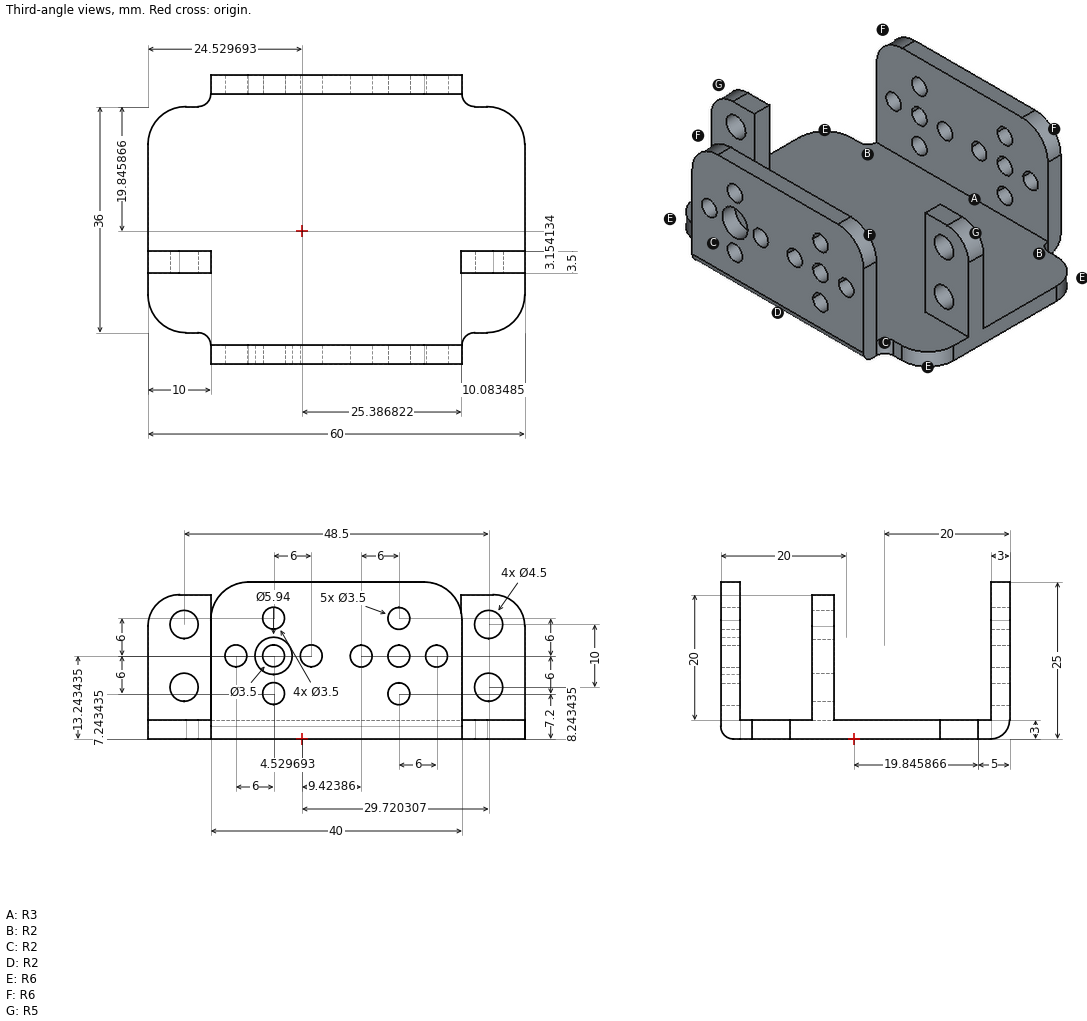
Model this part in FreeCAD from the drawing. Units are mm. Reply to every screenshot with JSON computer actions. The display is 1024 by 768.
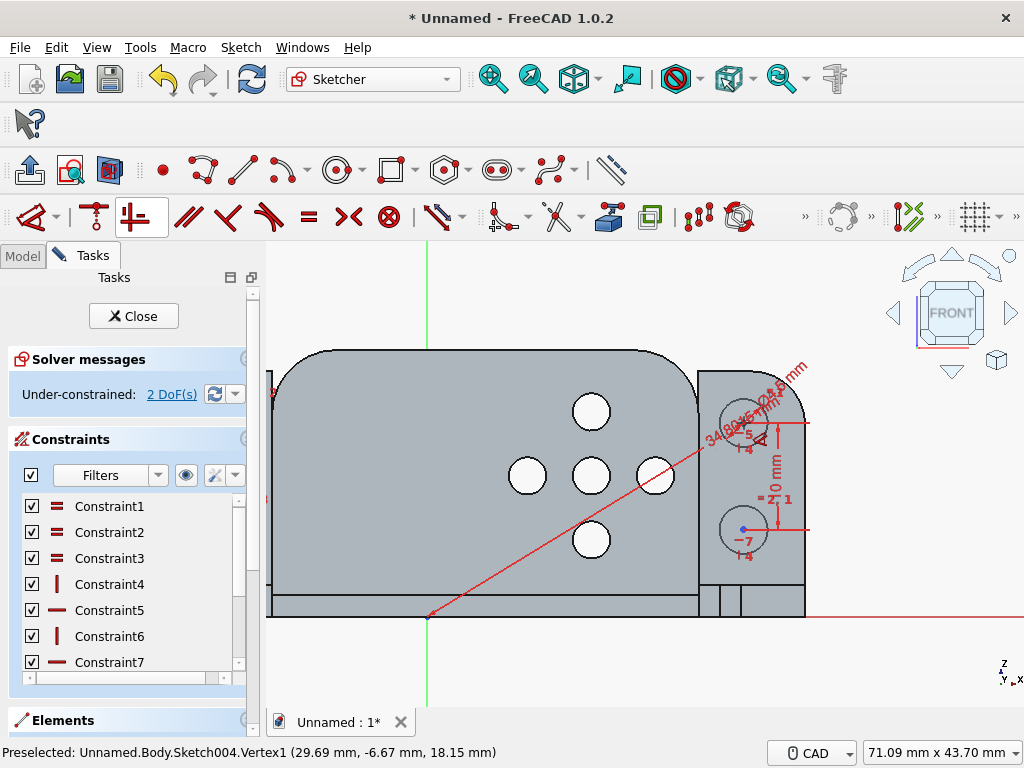
{"action": "scroll", "coordinate": [762, 406], "scroll_direction": "down", "scroll_amount": 2}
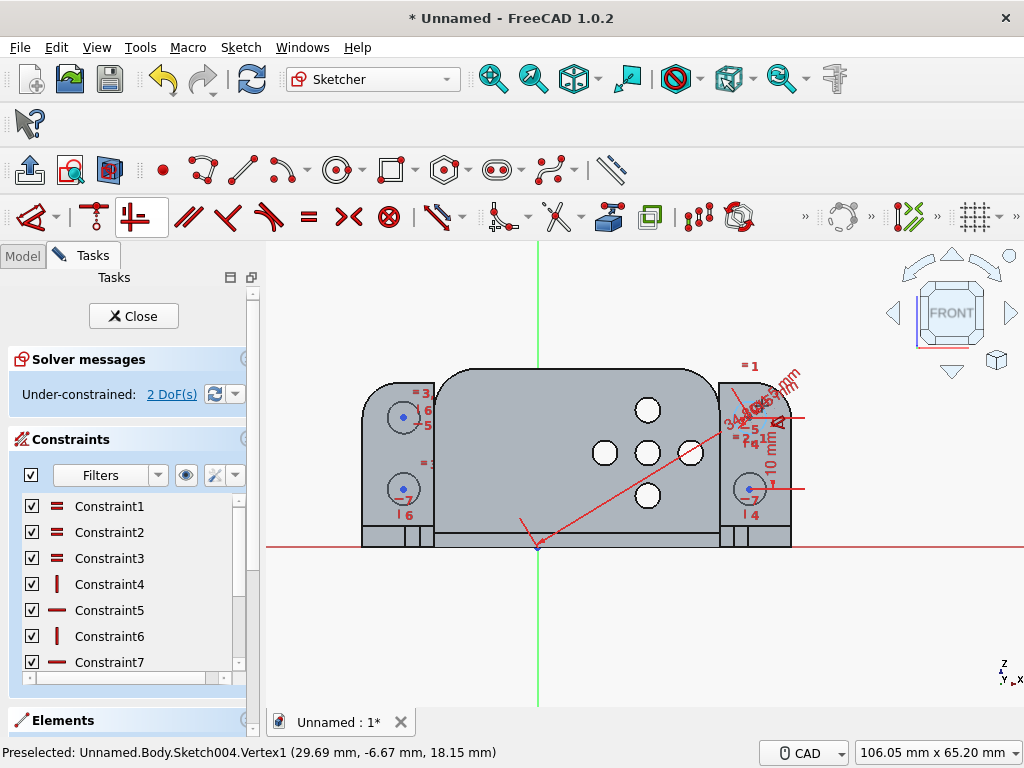
{"action": "left_click", "coordinate": [404, 418]}
{"action": "left_click", "coordinate": [577, 384]}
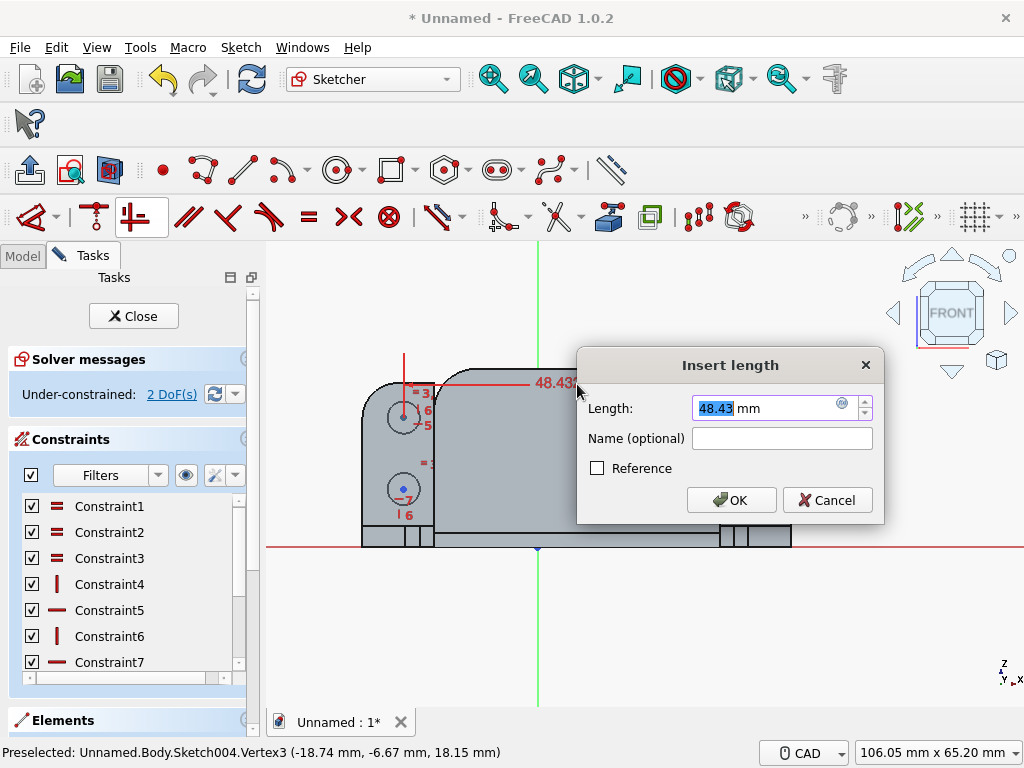
{"action": "type", "text": "48.5"}
{"action": "key", "text": "Return"}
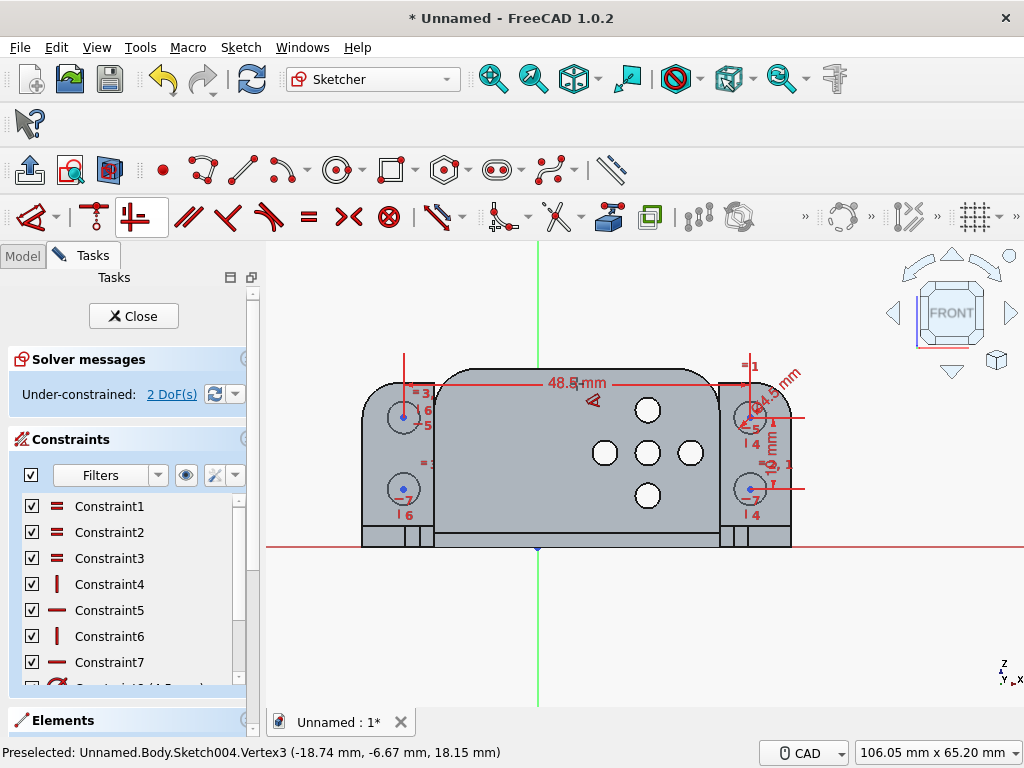
{"action": "left_click", "coordinate": [750, 489]}
{"action": "left_click", "coordinate": [784, 518]}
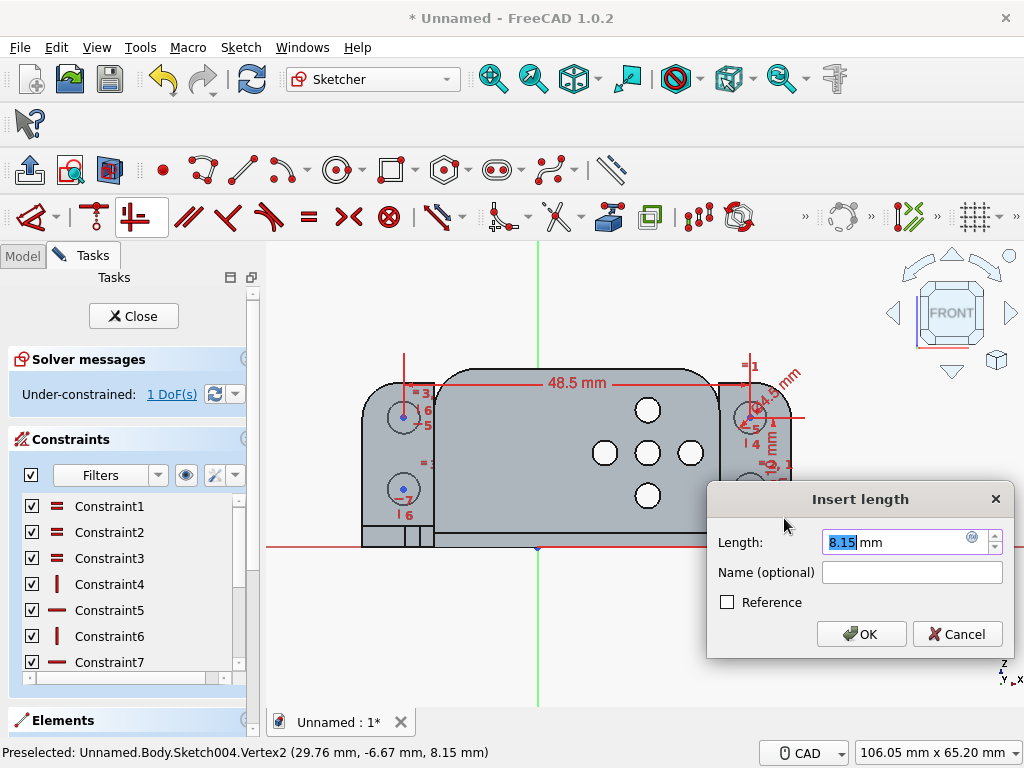
{"action": "type", "text": "8.243435"}
{"action": "key", "text": "Return"}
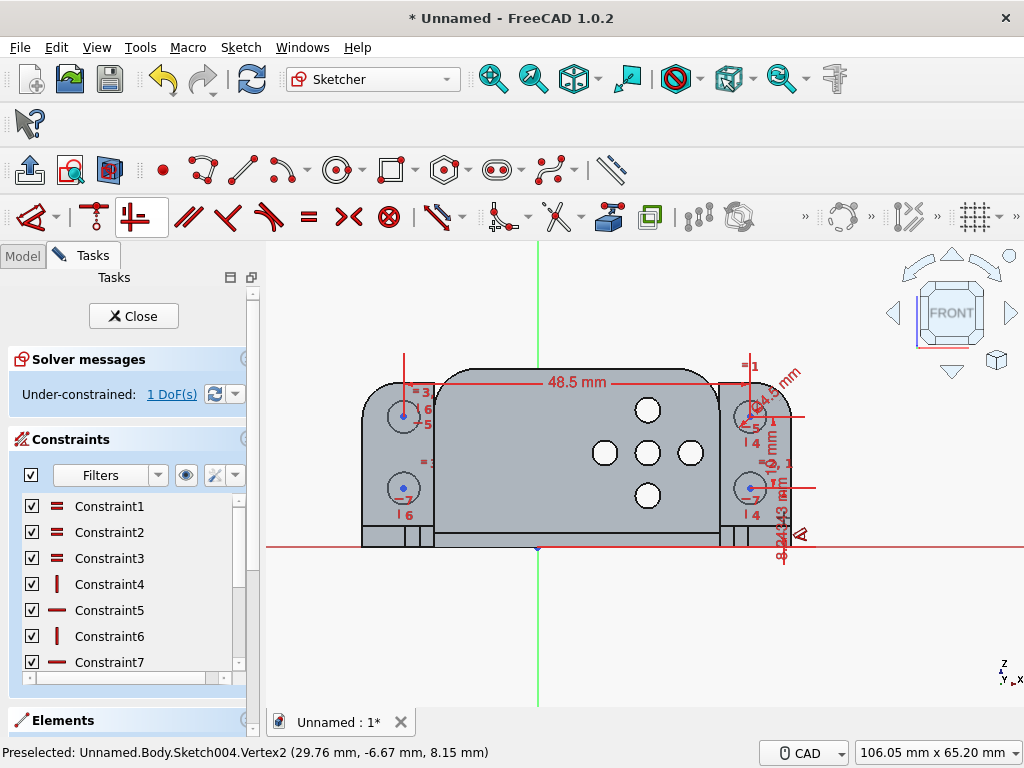
{"action": "left_click", "coordinate": [750, 417]}
{"action": "left_click", "coordinate": [644, 581]}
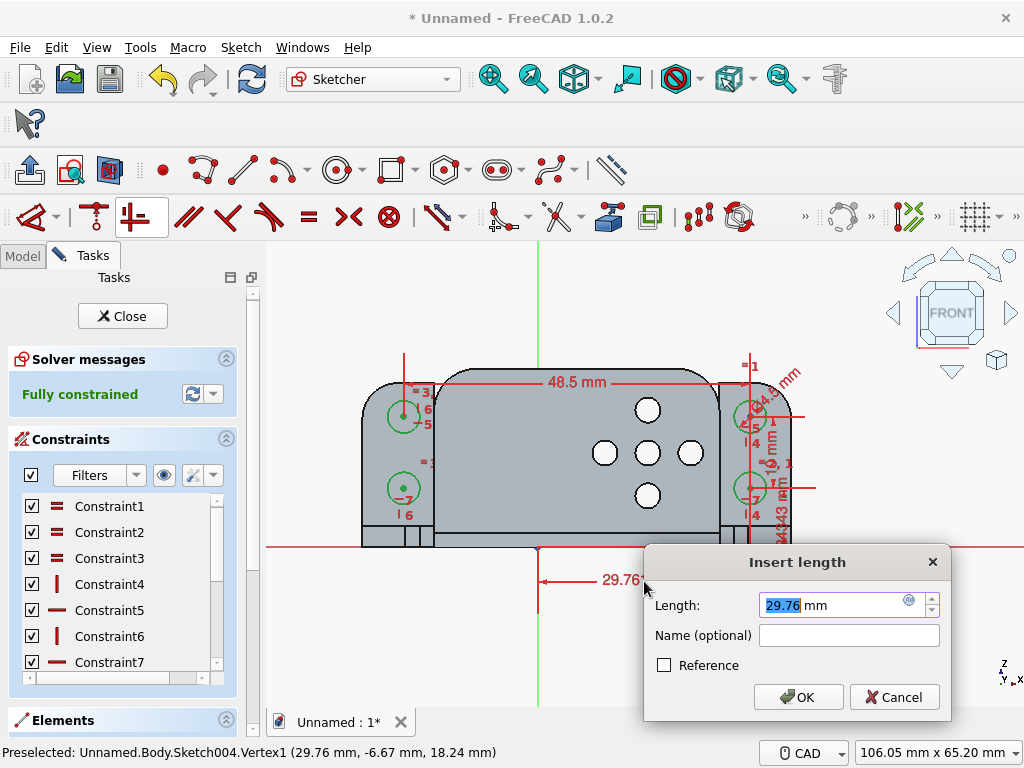
{"action": "type", "text": "29.720307"}
{"action": "key", "text": "Return"}
{"action": "key", "text": "Escape"}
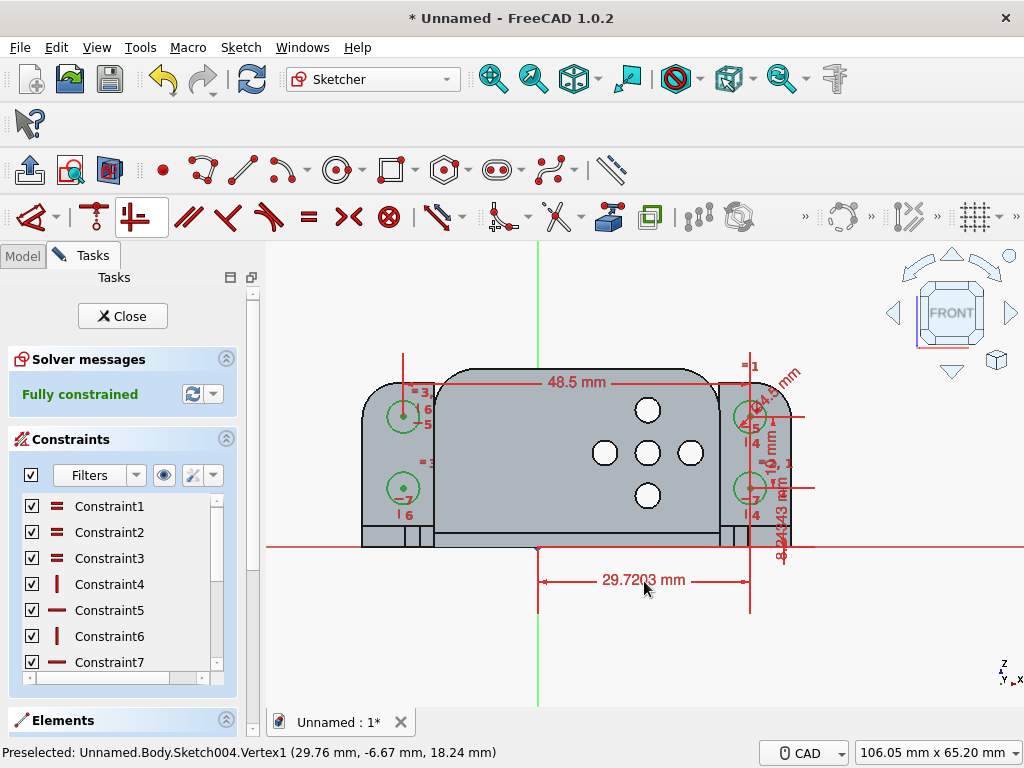
{"action": "left_click", "coordinate": [123, 316]}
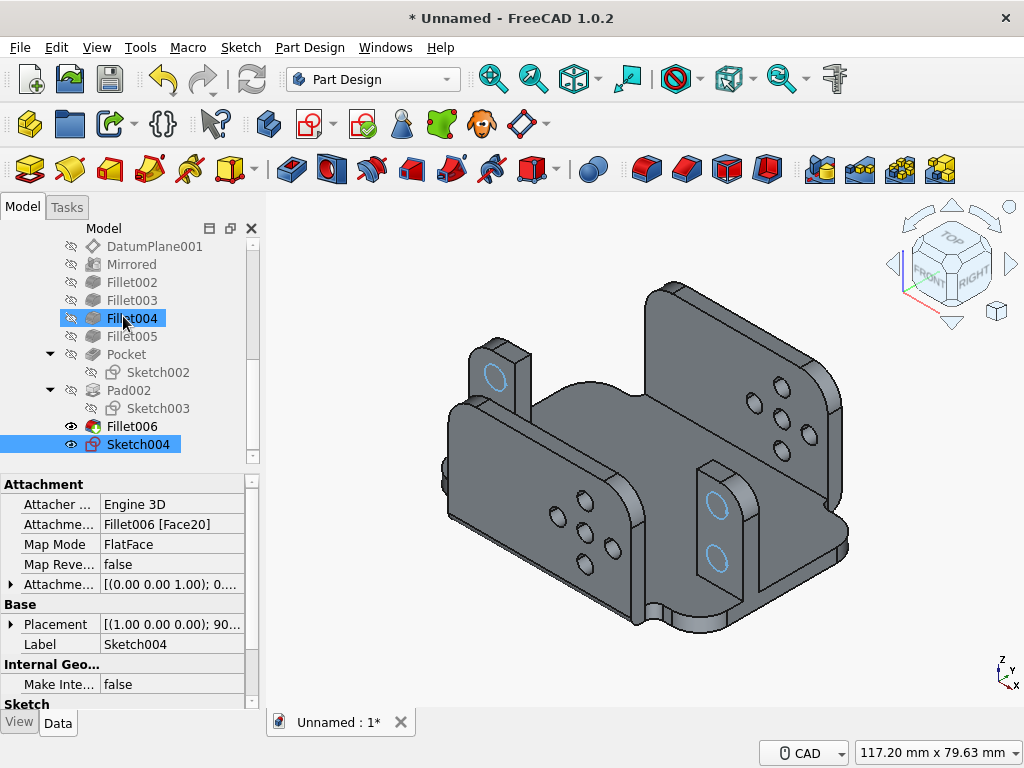
{"action": "left_click", "coordinate": [292, 170]}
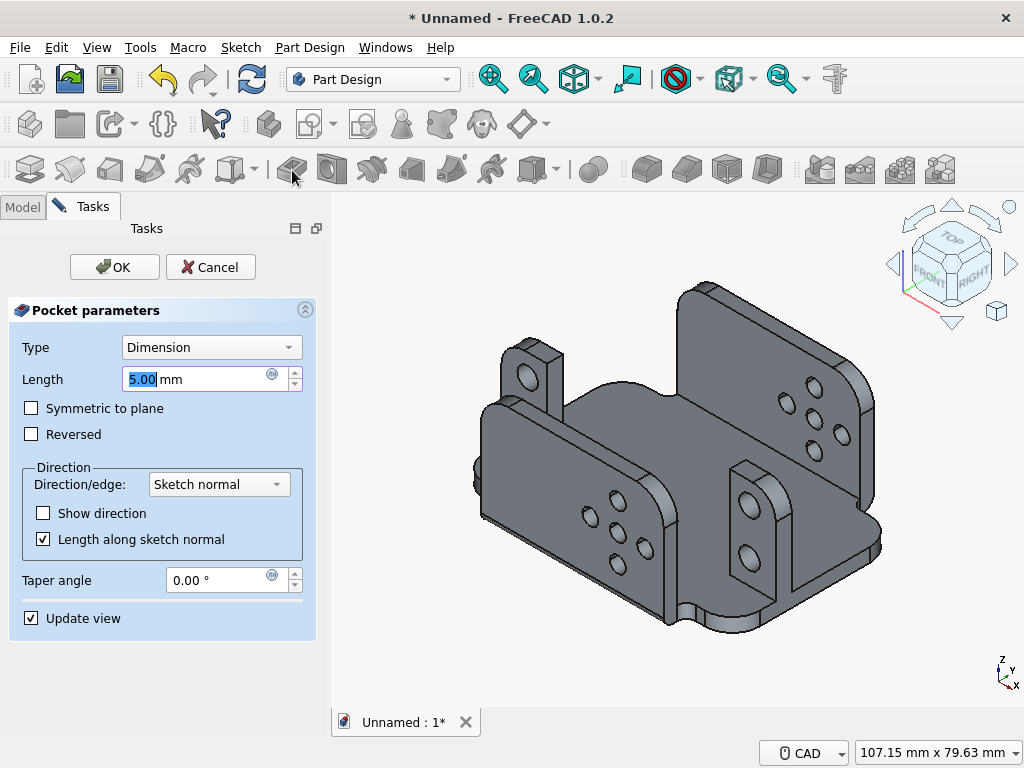
{"action": "left_click", "coordinate": [212, 348]}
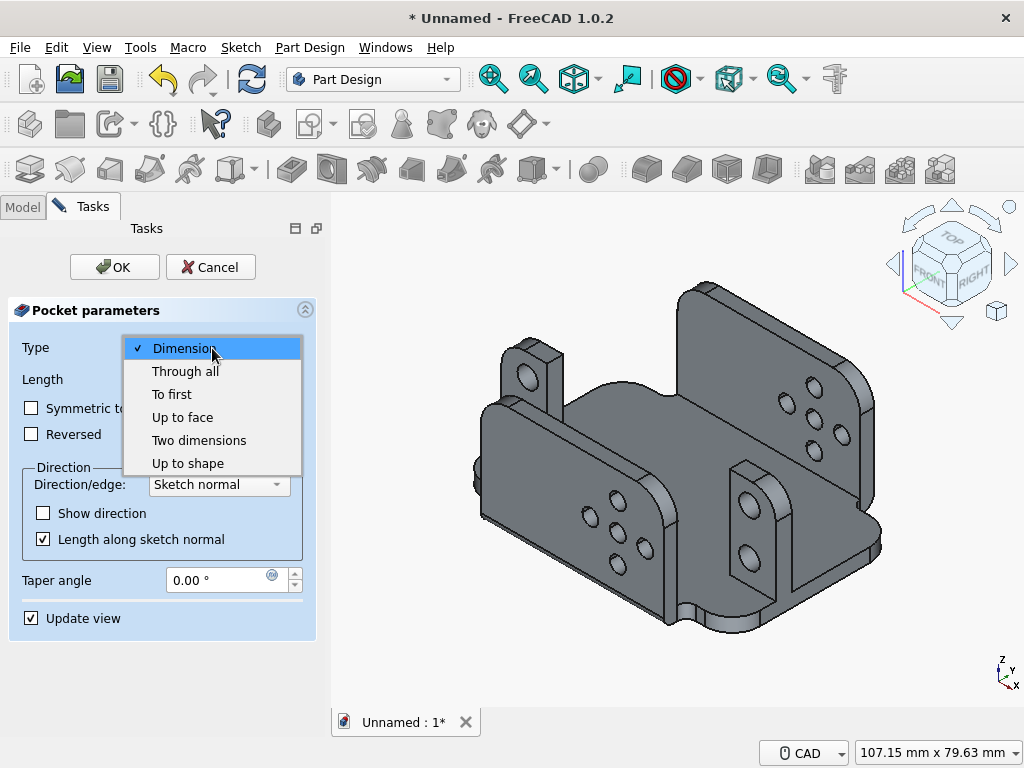
{"action": "left_click", "coordinate": [212, 372]}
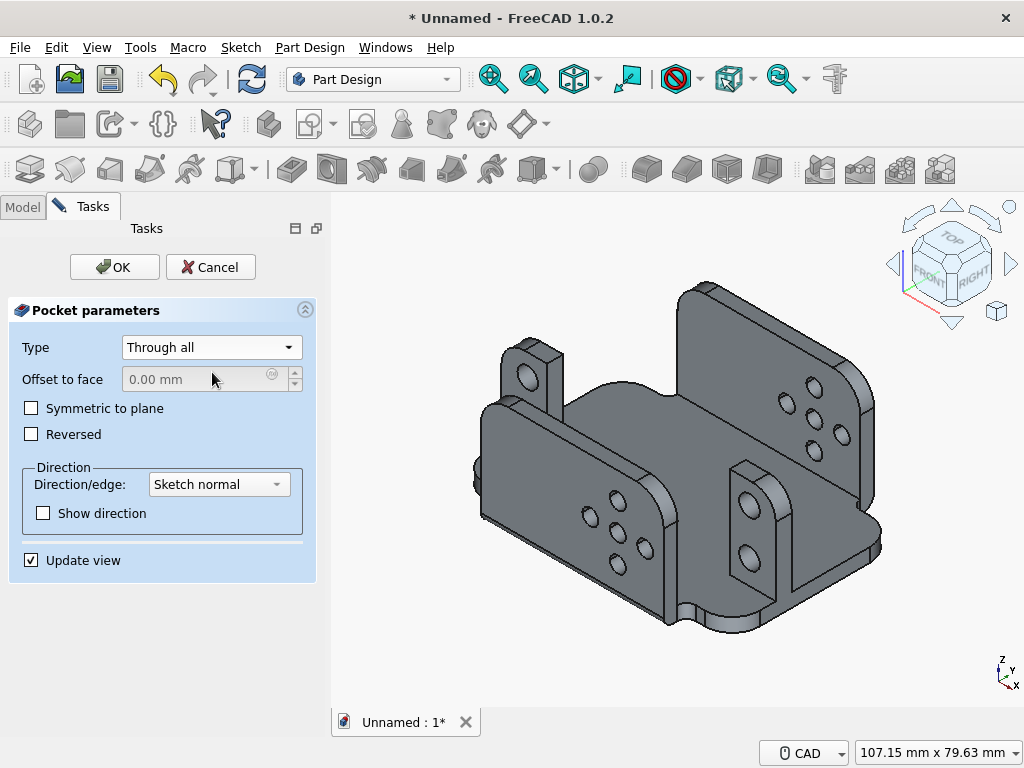
{"action": "left_click", "coordinate": [115, 267]}